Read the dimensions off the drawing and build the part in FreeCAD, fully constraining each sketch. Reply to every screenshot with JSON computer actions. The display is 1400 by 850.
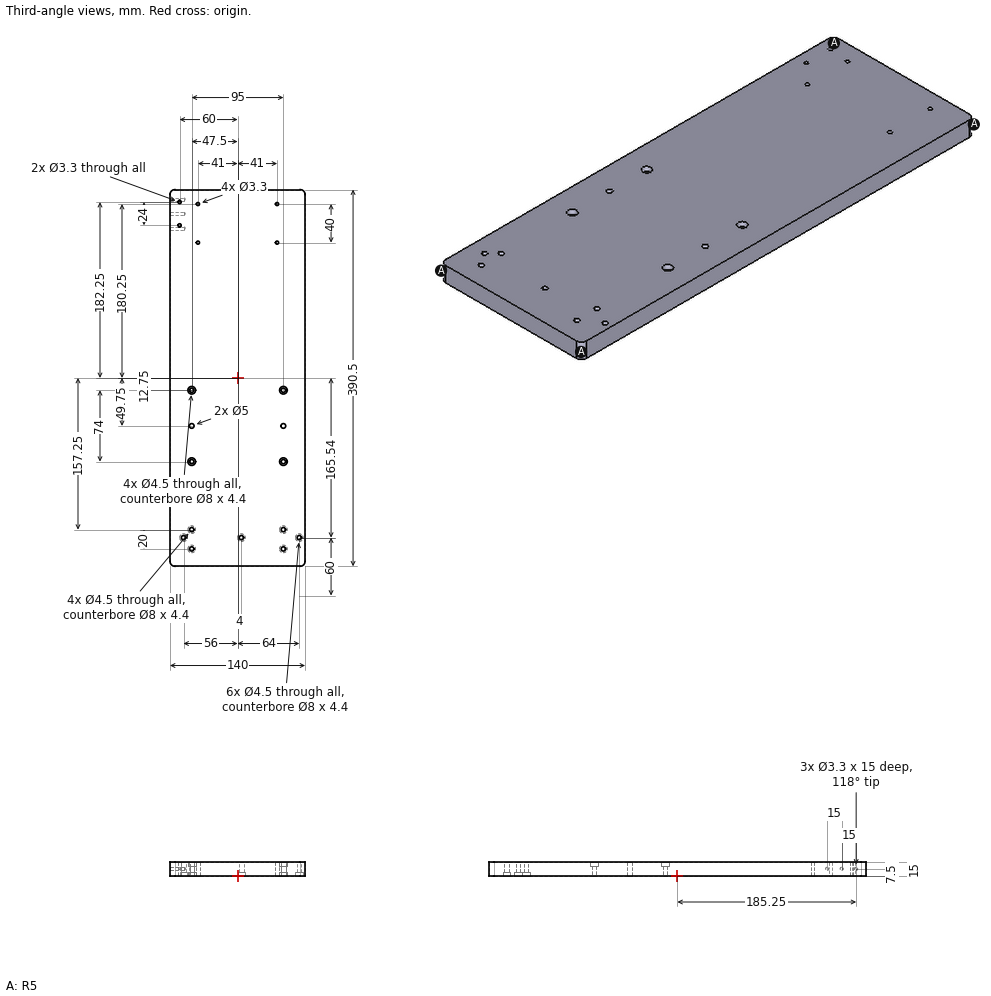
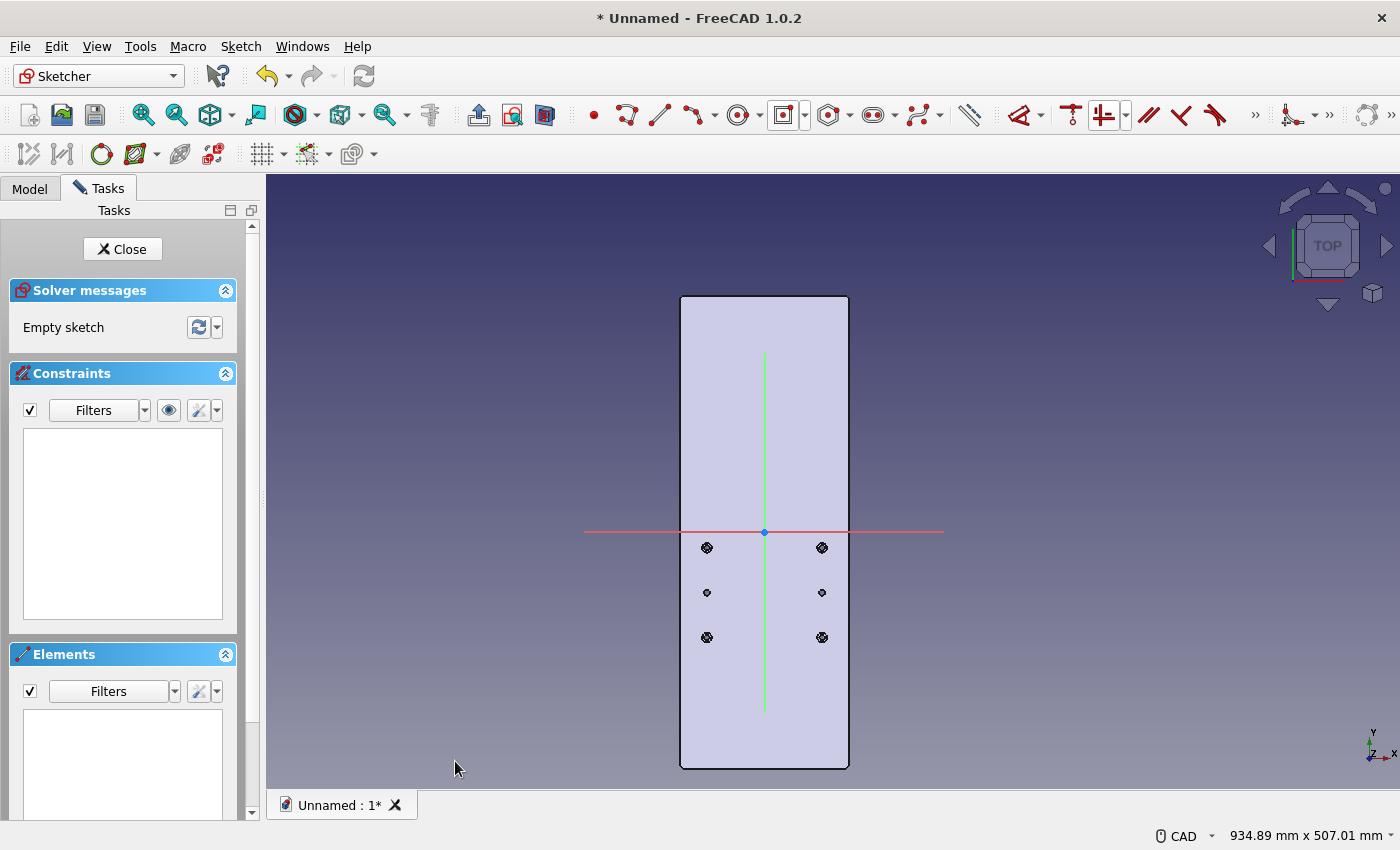
{"action": "scroll", "coordinate": [765, 350], "scroll_direction": "up", "scroll_amount": 3}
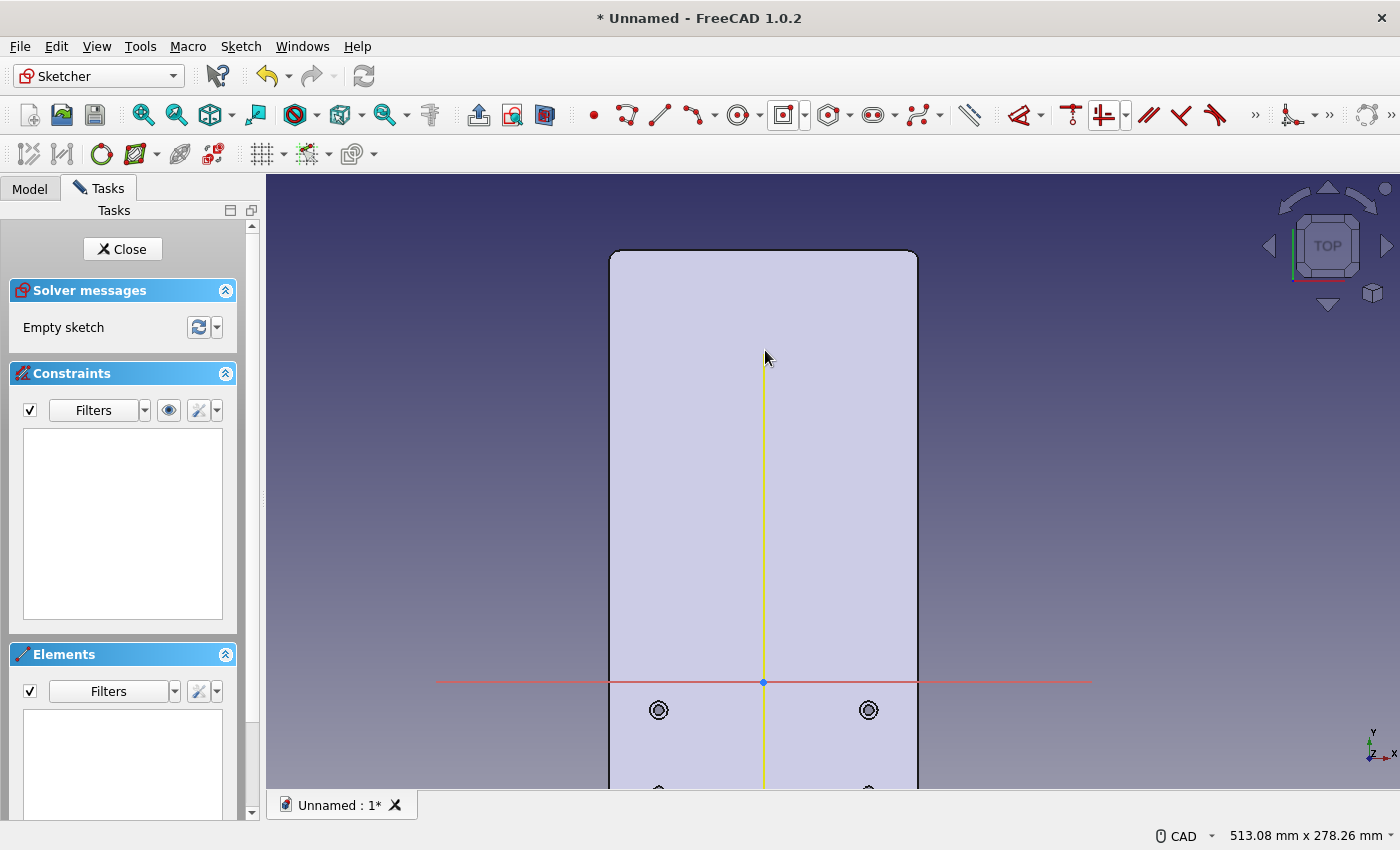
{"action": "left_click", "coordinate": [738, 116]}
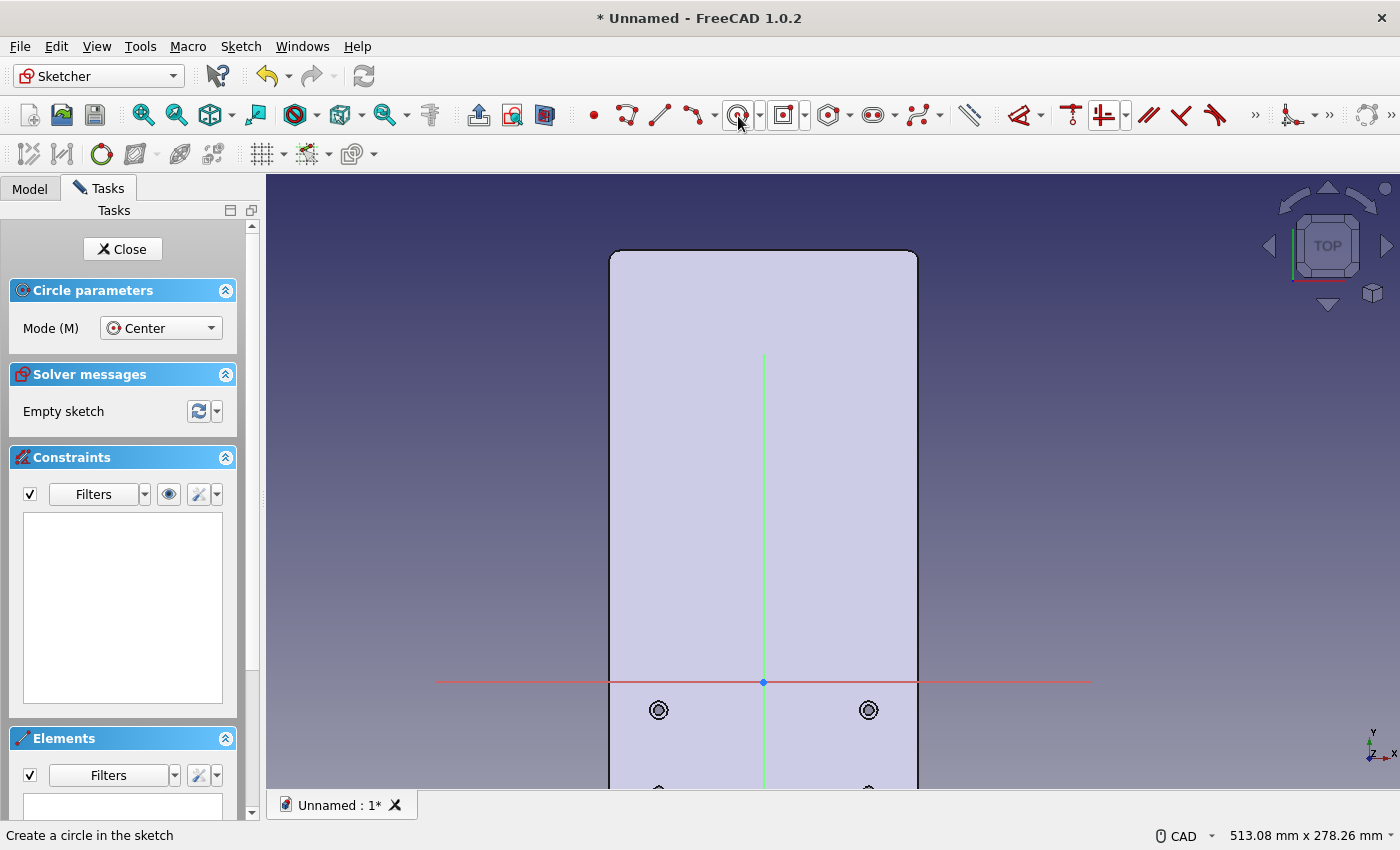
{"action": "scroll", "coordinate": [673, 284], "scroll_direction": "up", "scroll_amount": 10}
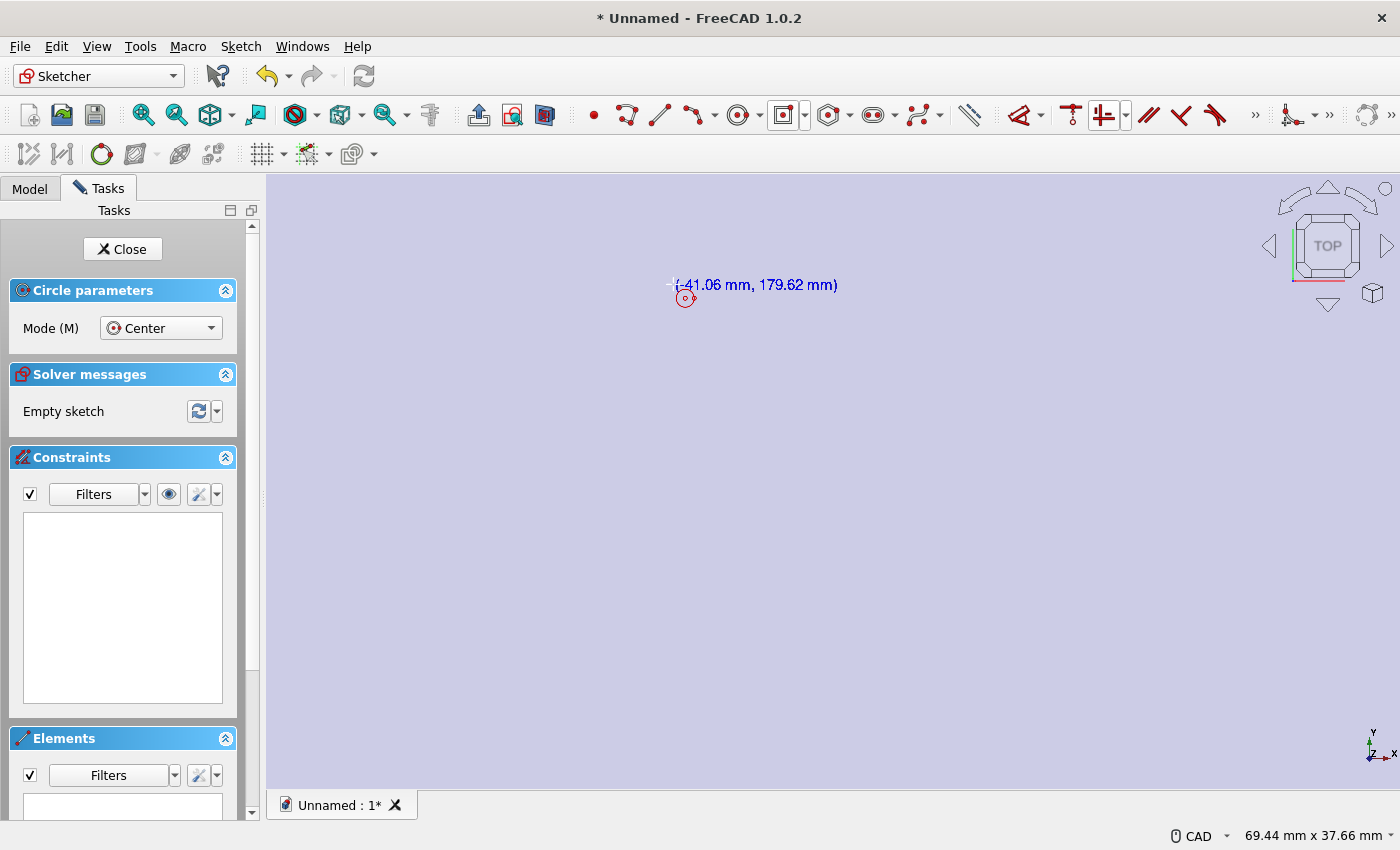
{"action": "scroll", "coordinate": [674, 285], "scroll_direction": "down", "scroll_amount": 10}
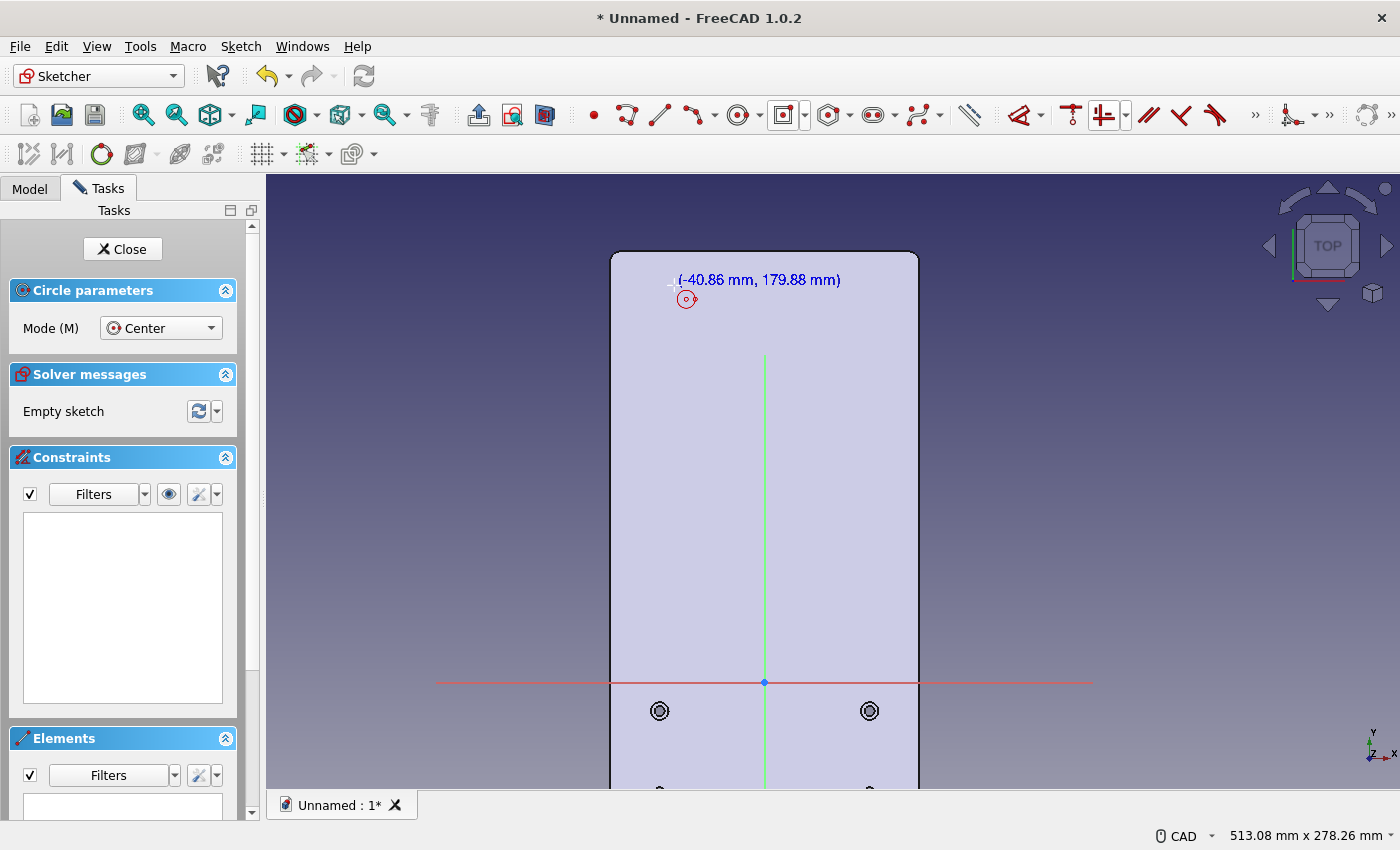
{"action": "left_click", "coordinate": [674, 284]}
{"action": "mouse_move", "coordinate": [677, 282]}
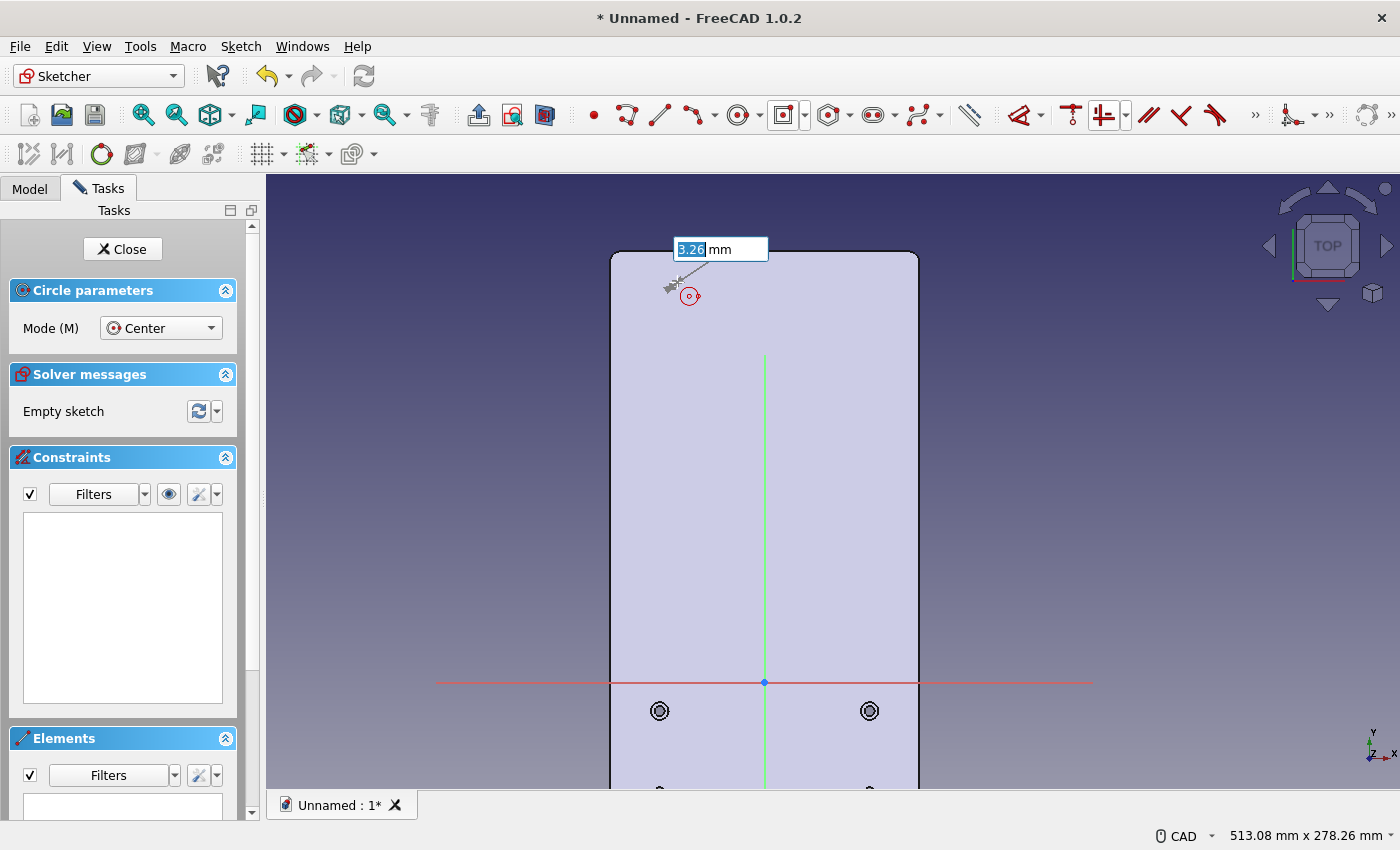
{"action": "type", "text": "3.3"}
{"action": "key", "text": "Return"}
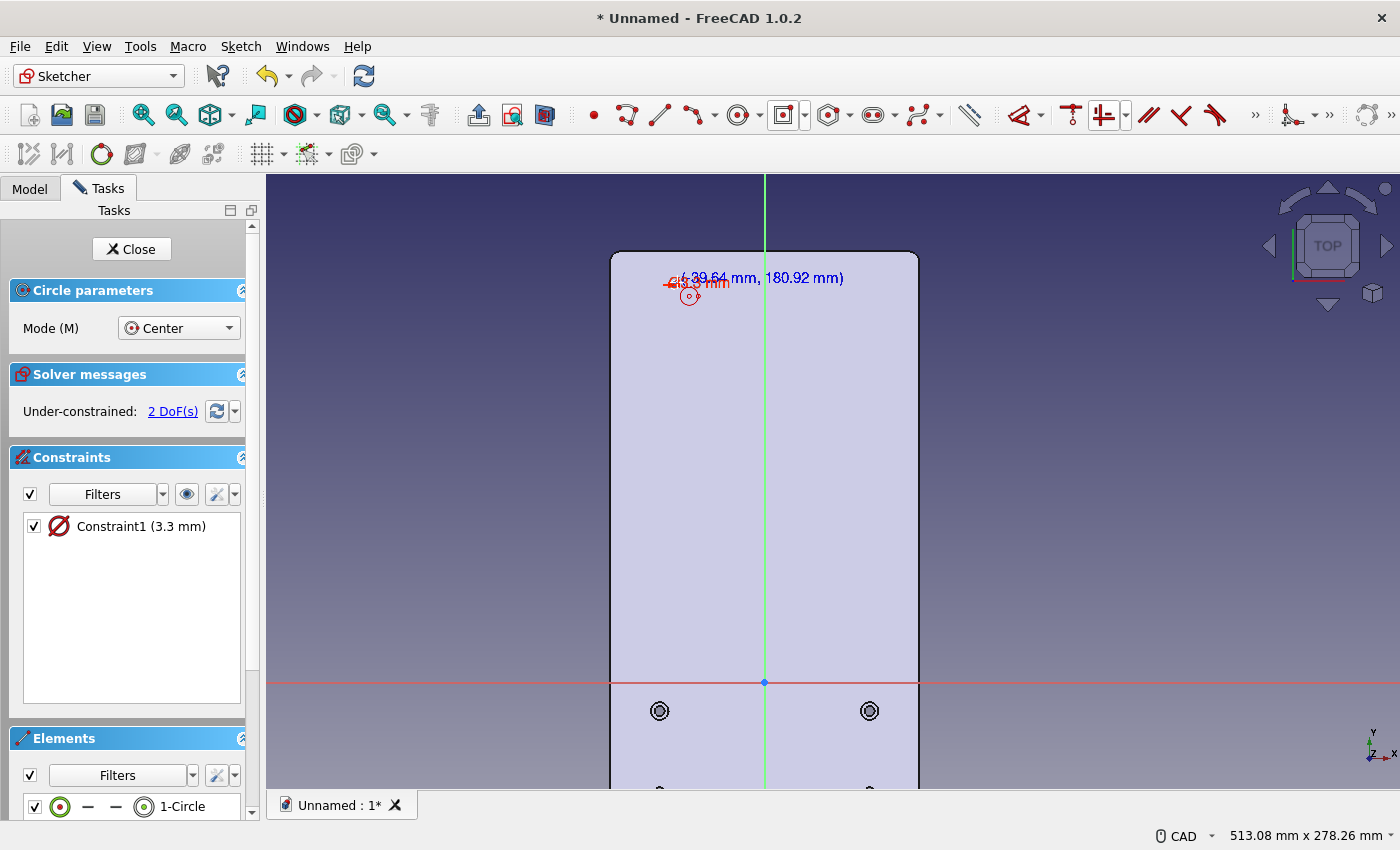
{"action": "scroll", "coordinate": [855, 284], "scroll_direction": "up", "scroll_amount": 10}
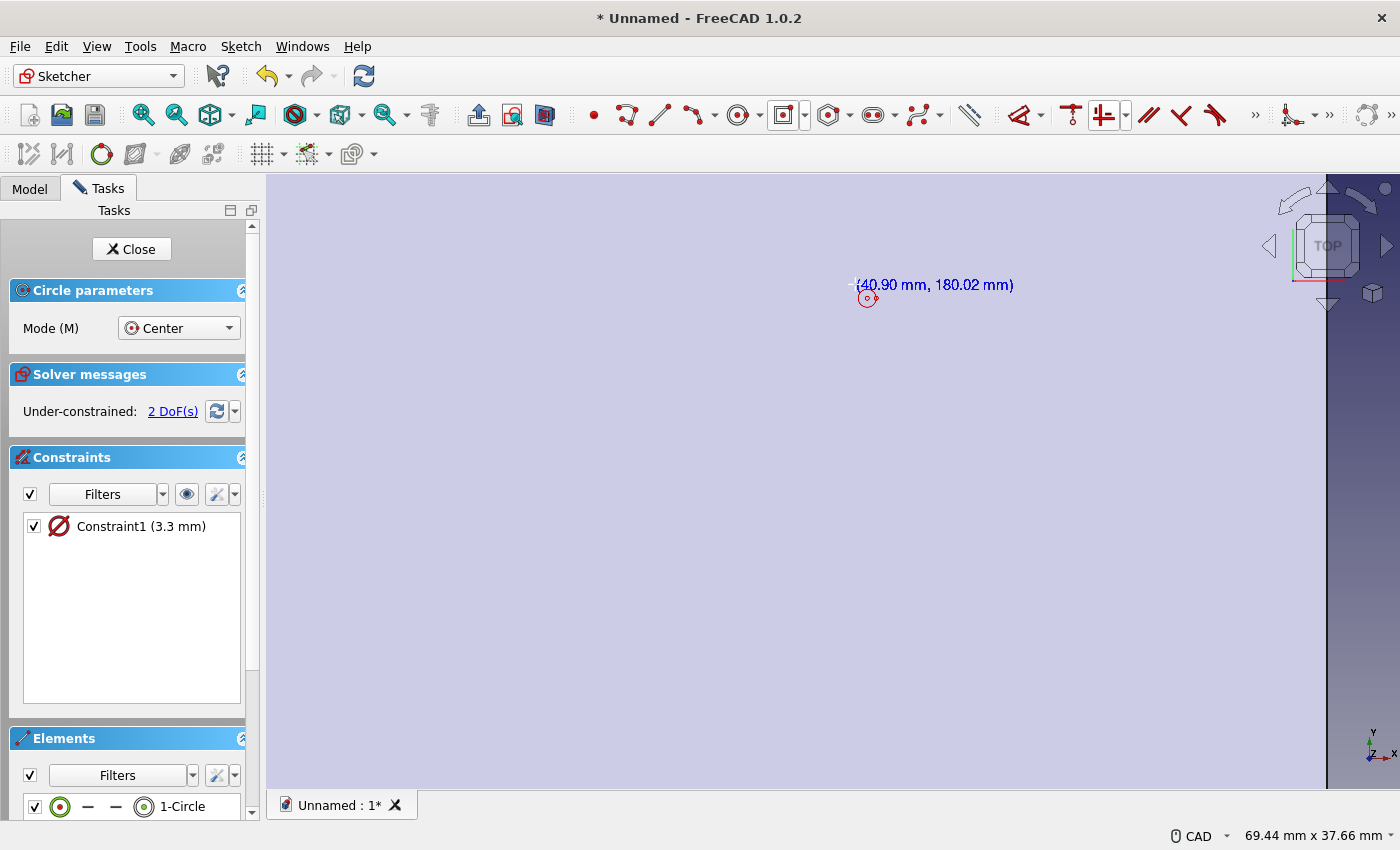
{"action": "scroll", "coordinate": [855, 284], "scroll_direction": "down", "scroll_amount": 10}